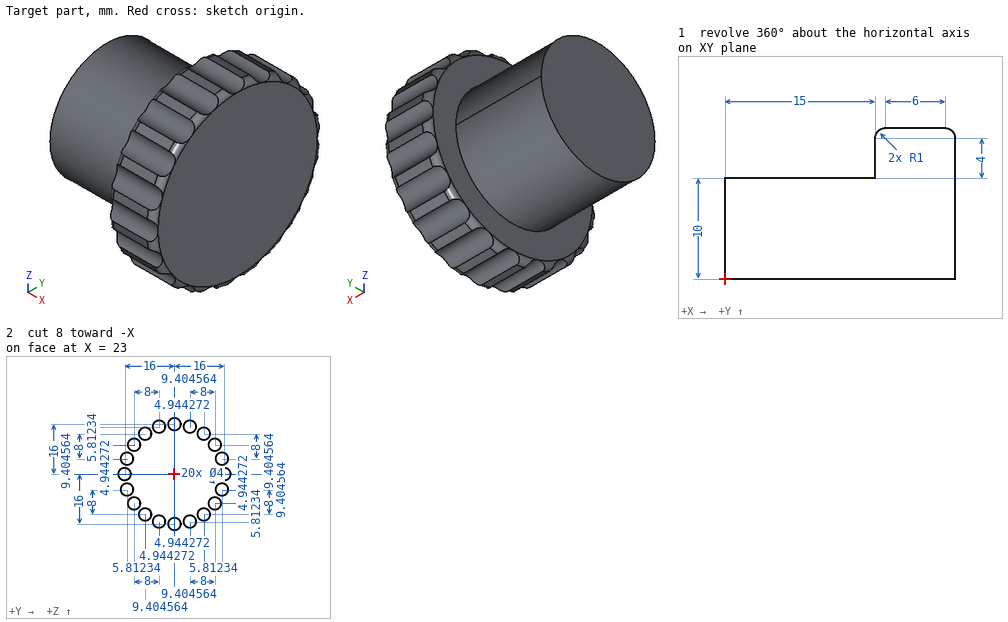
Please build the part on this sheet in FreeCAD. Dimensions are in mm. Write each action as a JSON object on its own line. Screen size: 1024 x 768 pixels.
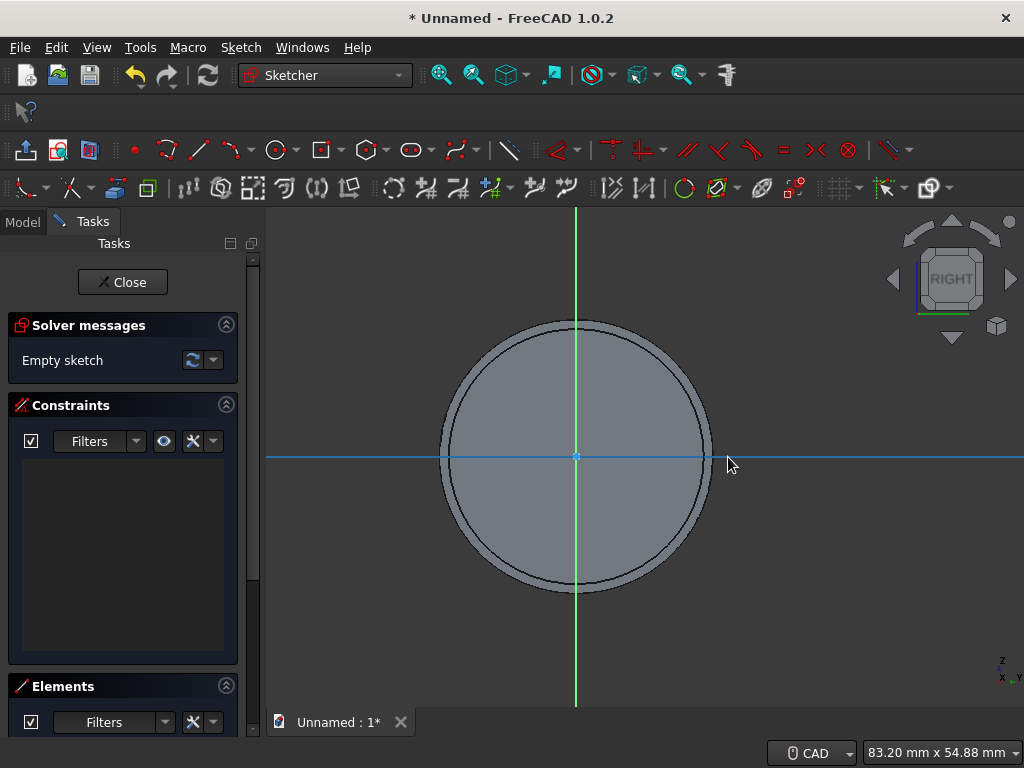
{"action": "left_click", "coordinate": [276, 150]}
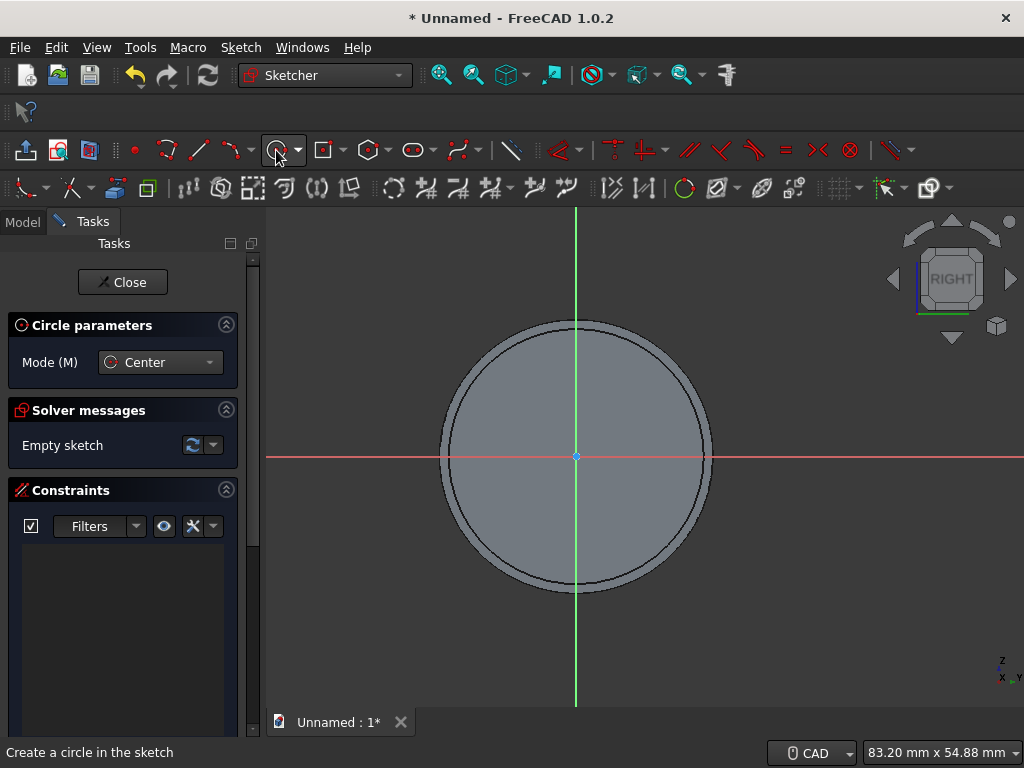
{"action": "scroll", "coordinate": [722, 457], "scroll_direction": "up", "scroll_amount": 2}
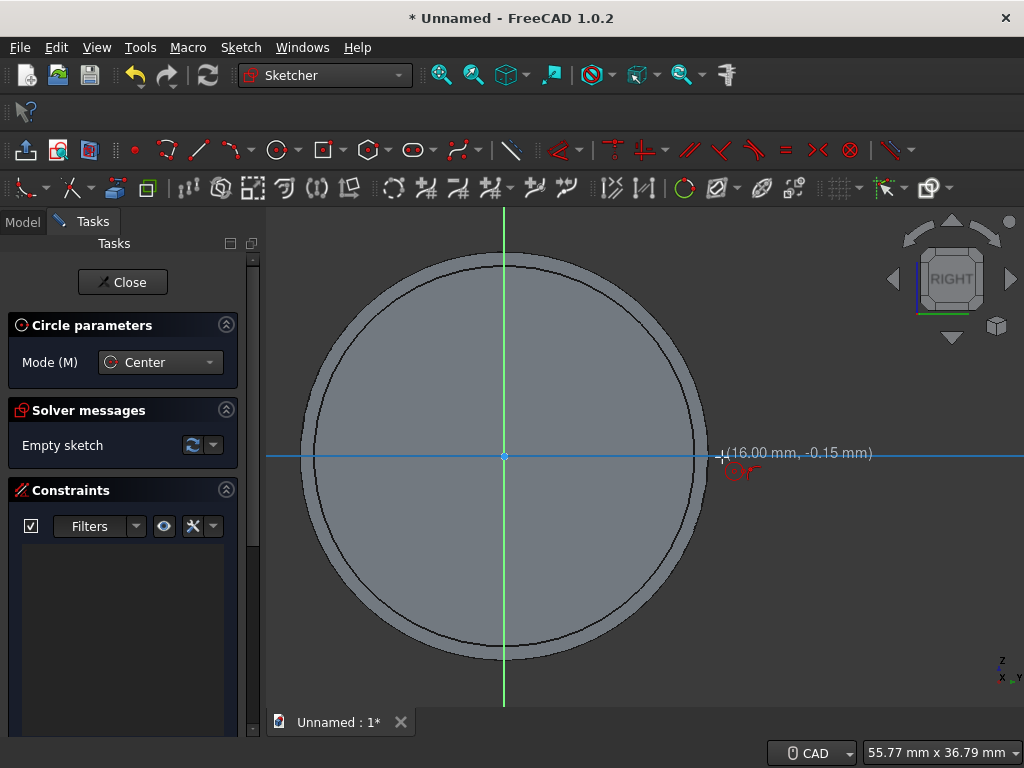
{"action": "left_click", "coordinate": [722, 456]}
{"action": "mouse_move", "coordinate": [741, 437]}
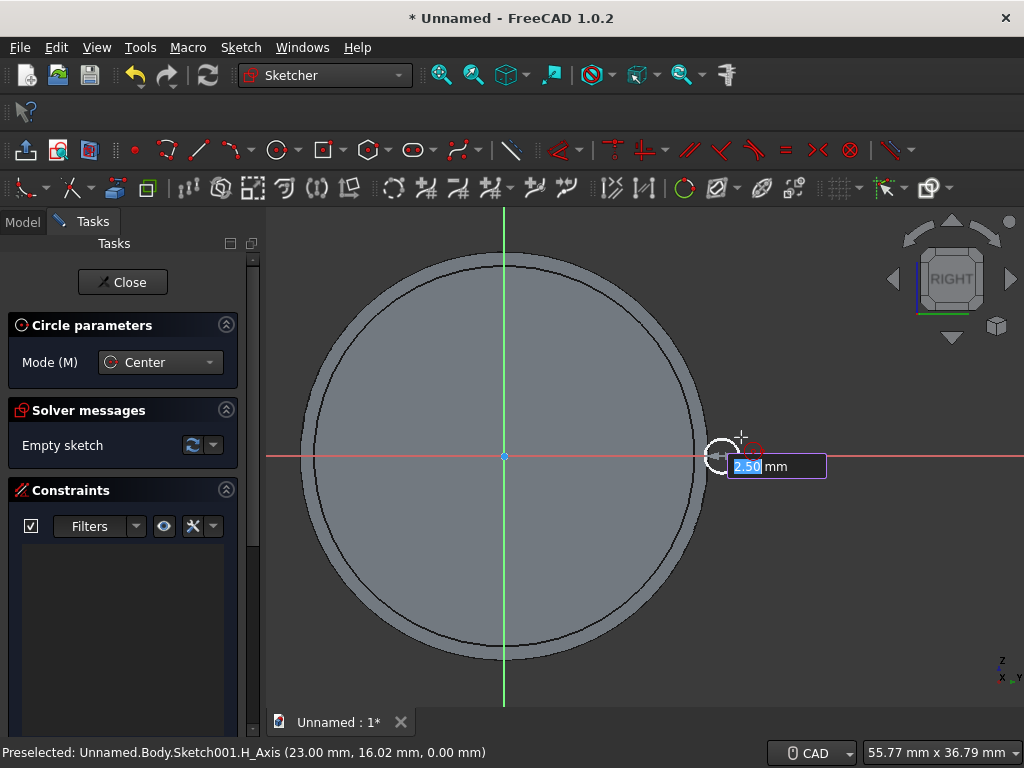
{"action": "type", "text": "4"}
{"action": "key", "text": "Return"}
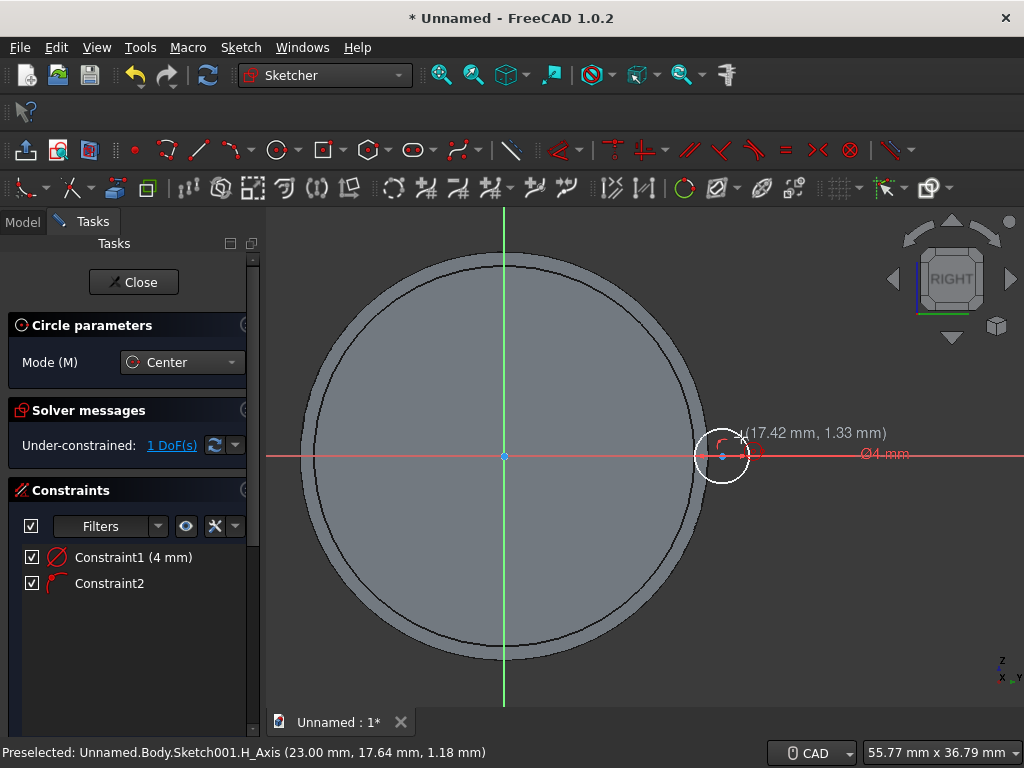
{"action": "left_click", "coordinate": [711, 523]}
{"action": "mouse_move", "coordinate": [730, 504]}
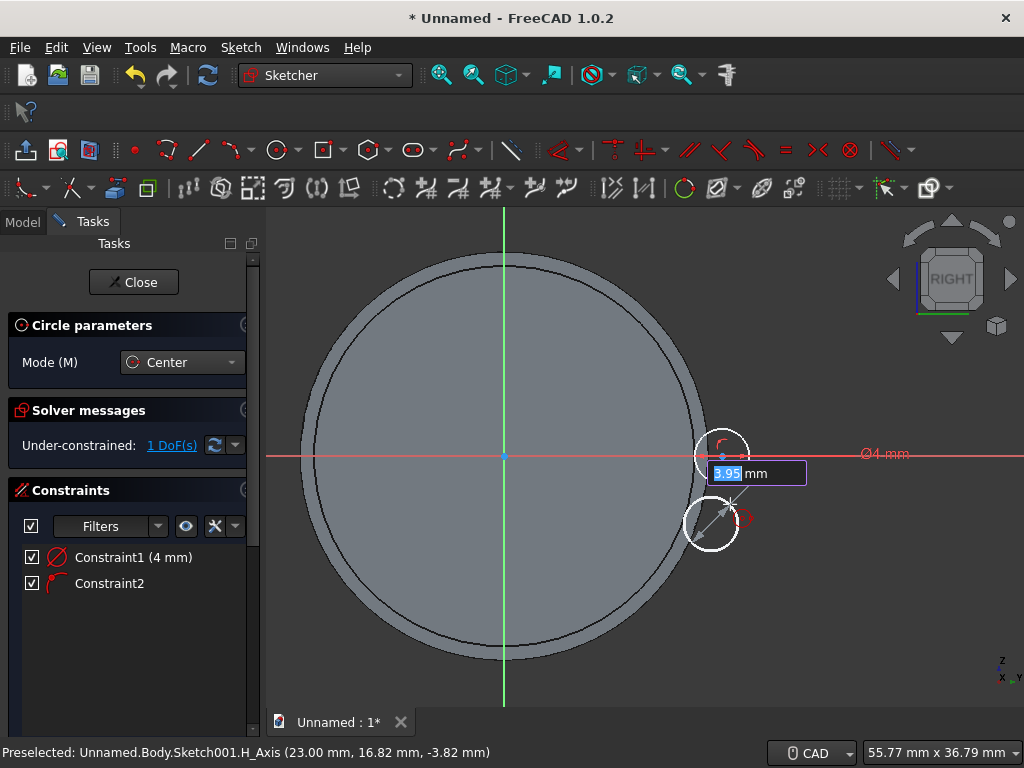
{"action": "type", "text": "4"}
{"action": "key", "text": "Return"}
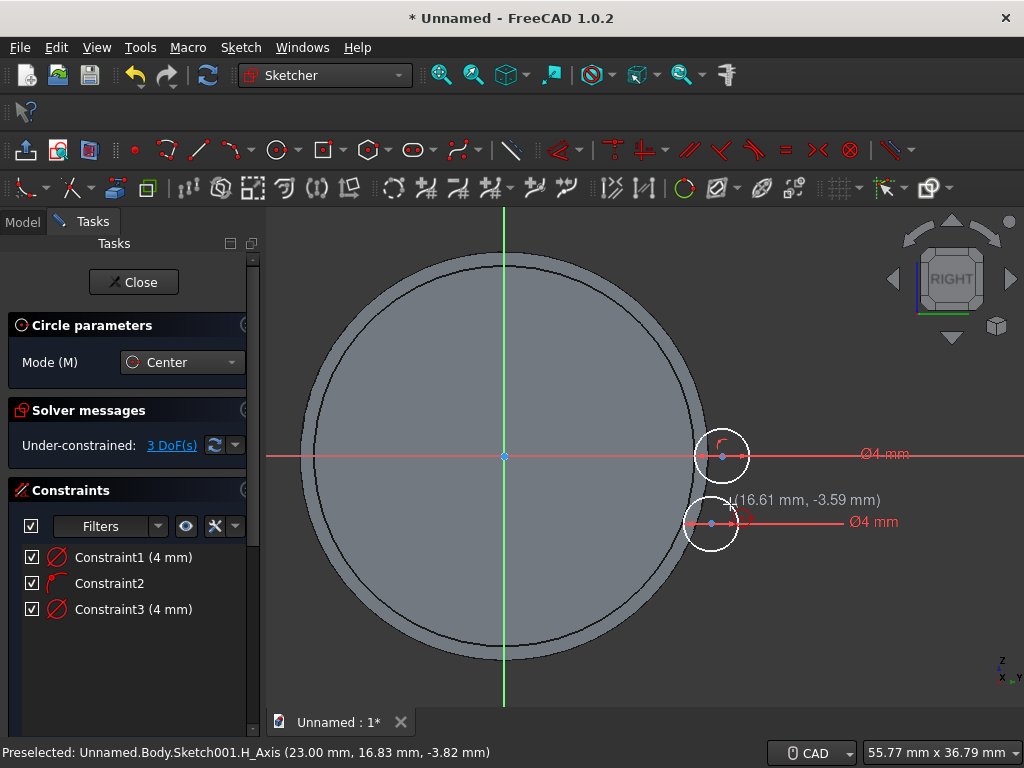
{"action": "left_click", "coordinate": [680, 584]}
{"action": "mouse_move", "coordinate": [699, 565]}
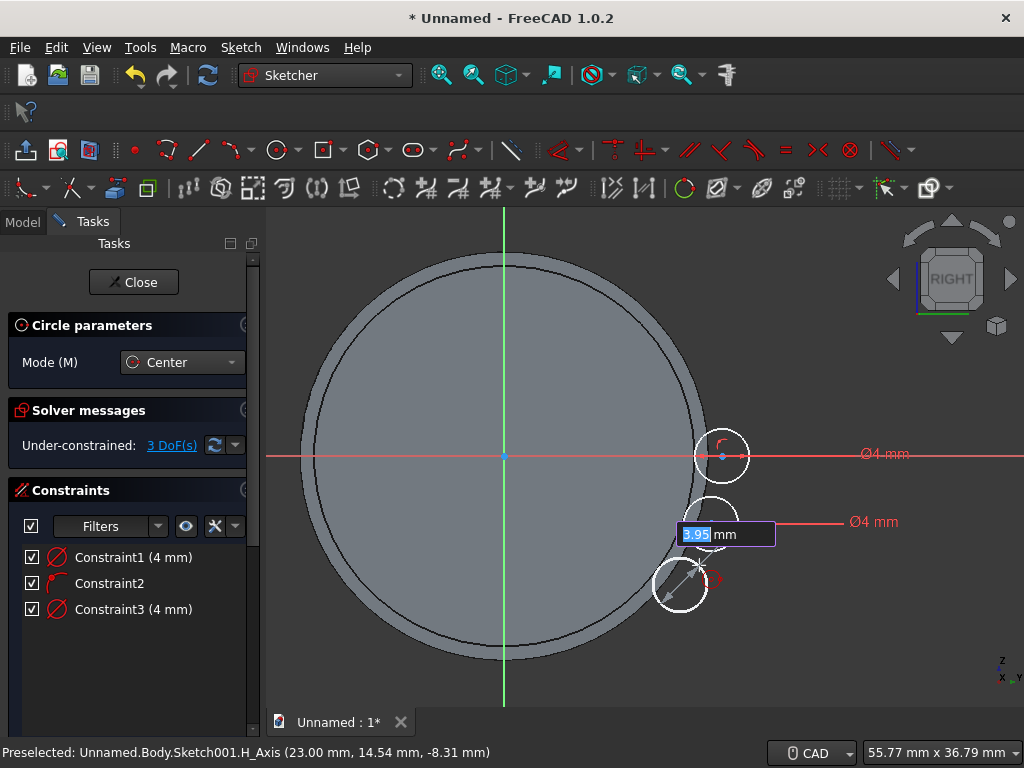
{"action": "type", "text": "4"}
{"action": "key", "text": "Return"}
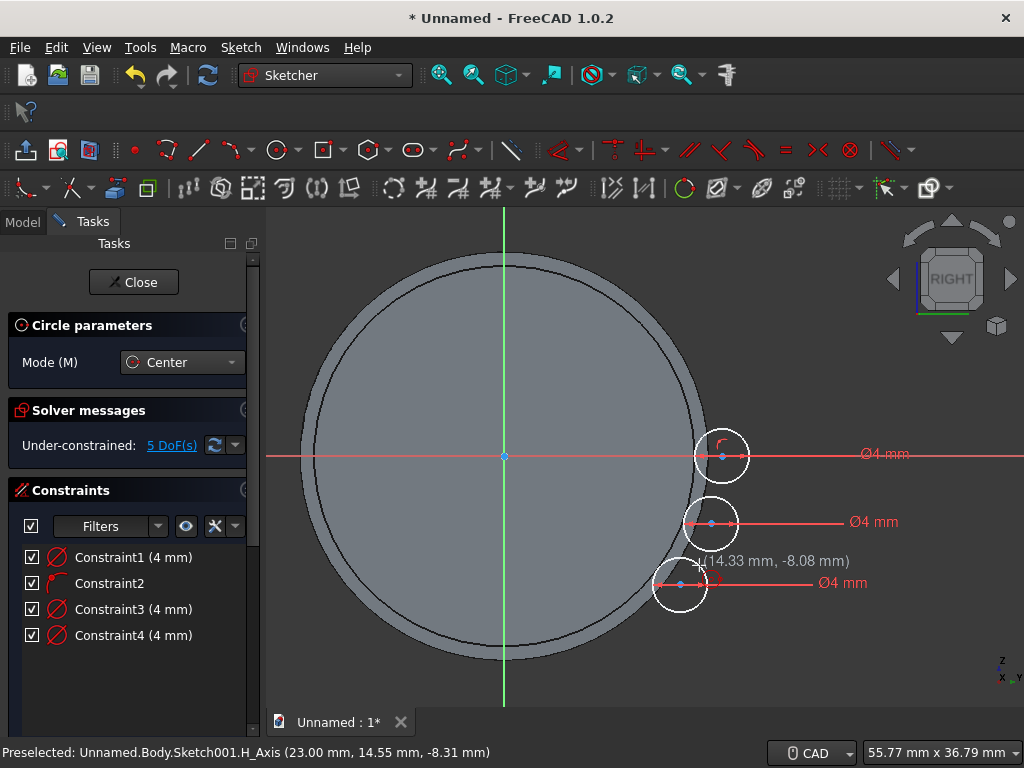
{"action": "left_click", "coordinate": [632, 632]}
{"action": "mouse_move", "coordinate": [613, 613]}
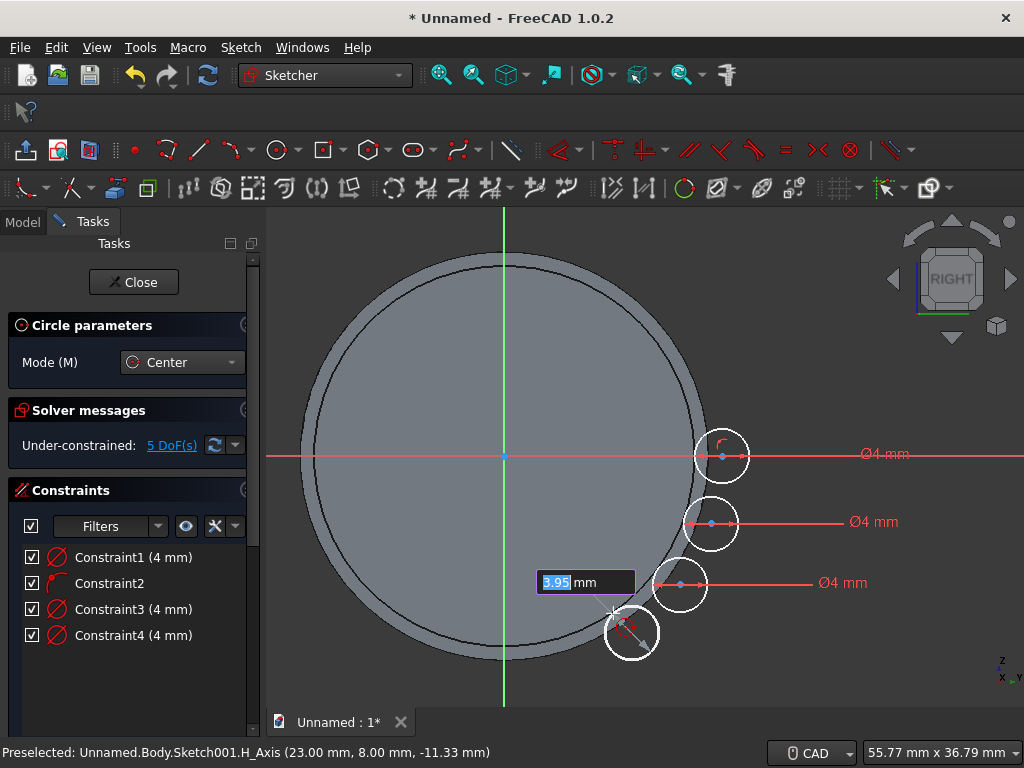
{"action": "type", "text": "4"}
{"action": "key", "text": "Return"}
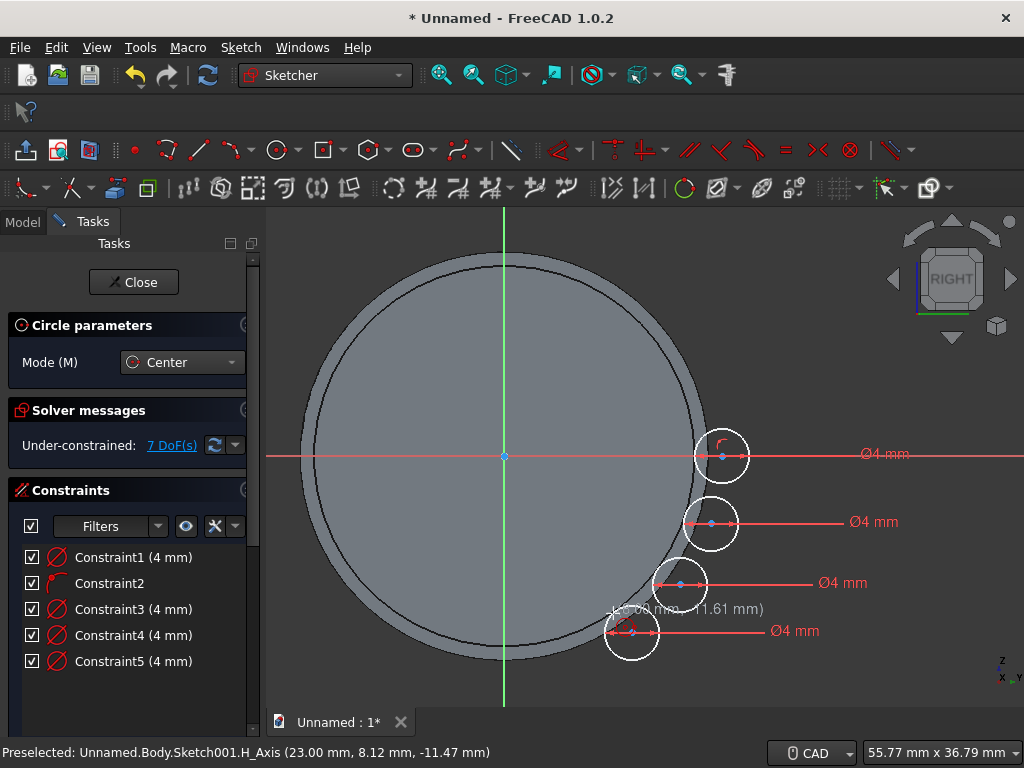
{"action": "left_click", "coordinate": [571, 663]}
{"action": "mouse_move", "coordinate": [591, 644]}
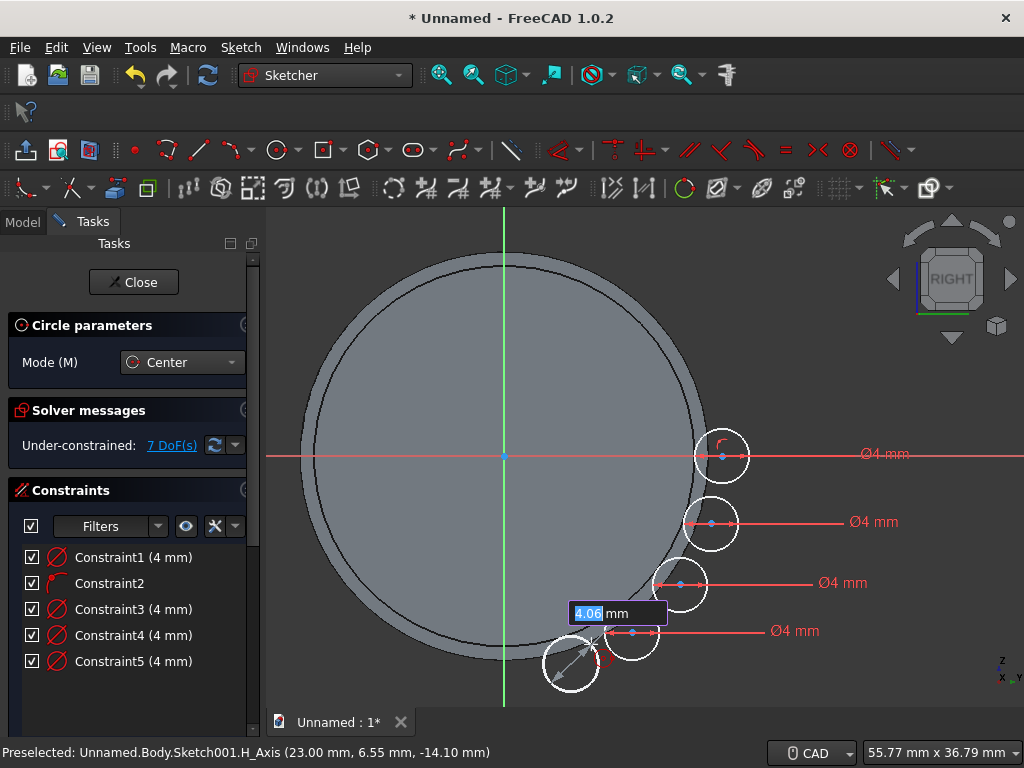
{"action": "type", "text": "4"}
{"action": "key", "text": "Return"}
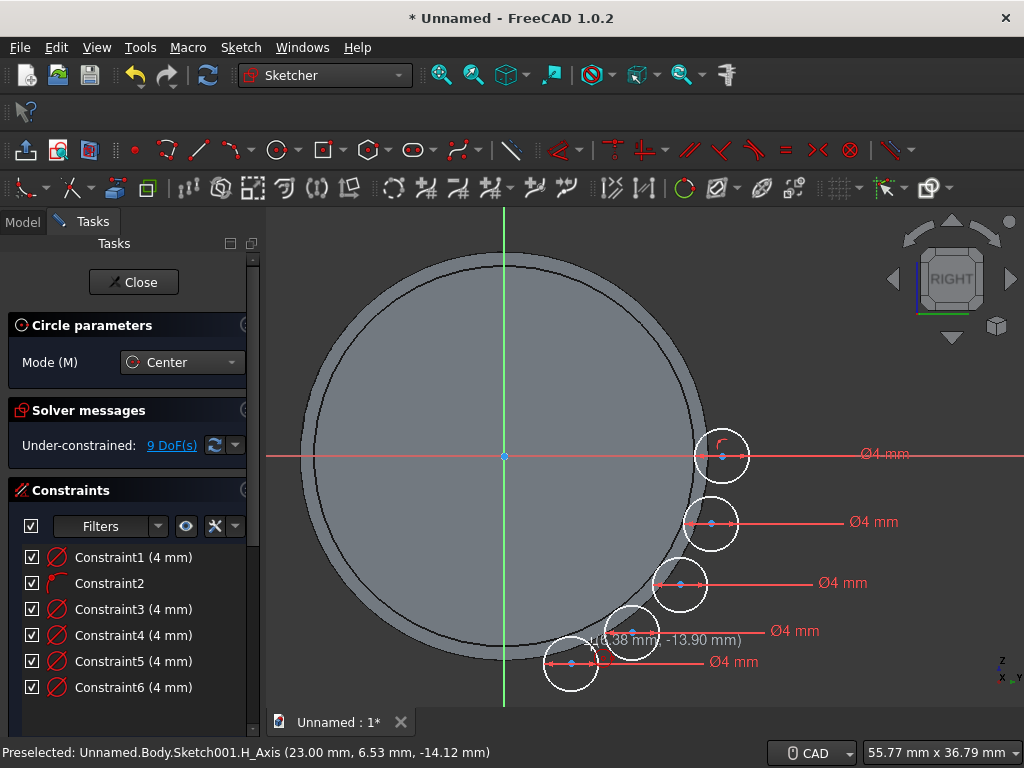
{"action": "left_click", "coordinate": [504, 674]}
{"action": "mouse_move", "coordinate": [524, 654]}